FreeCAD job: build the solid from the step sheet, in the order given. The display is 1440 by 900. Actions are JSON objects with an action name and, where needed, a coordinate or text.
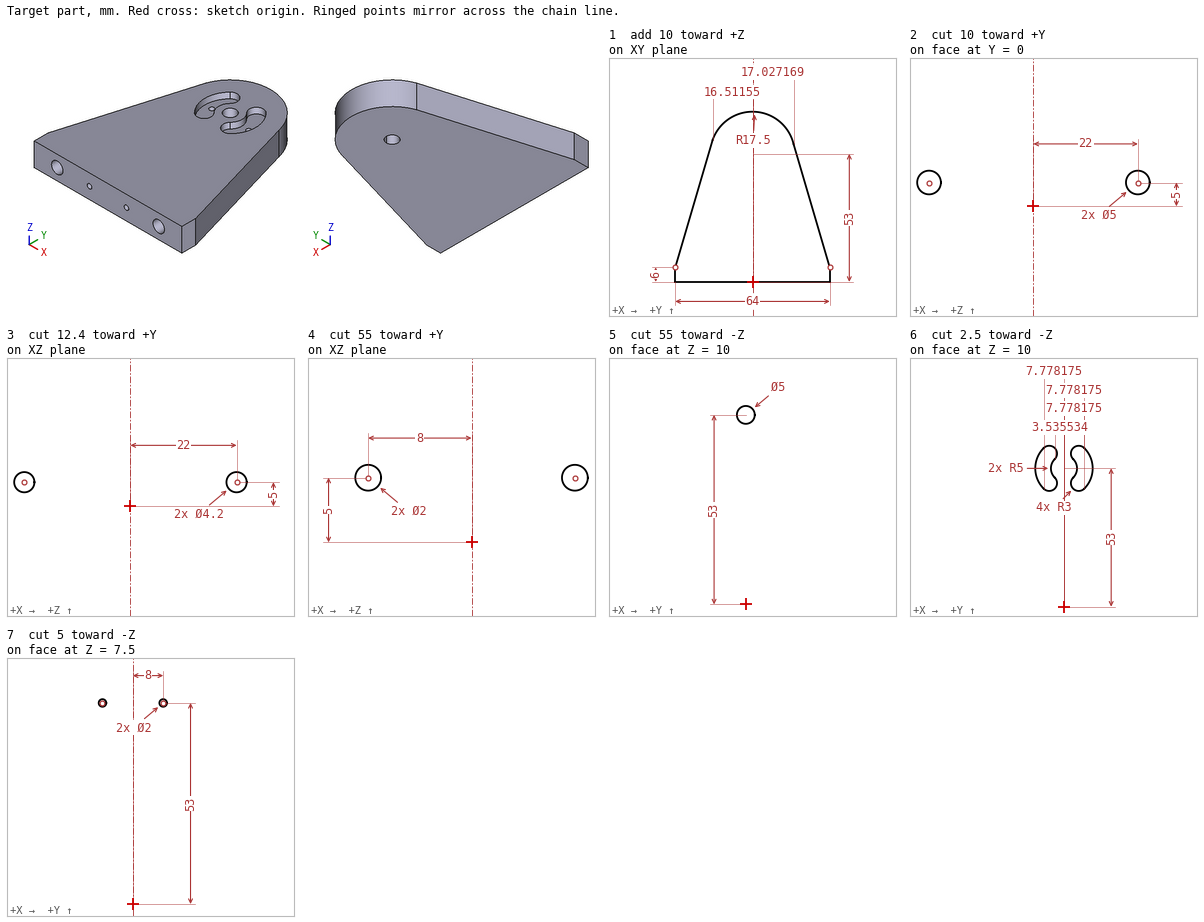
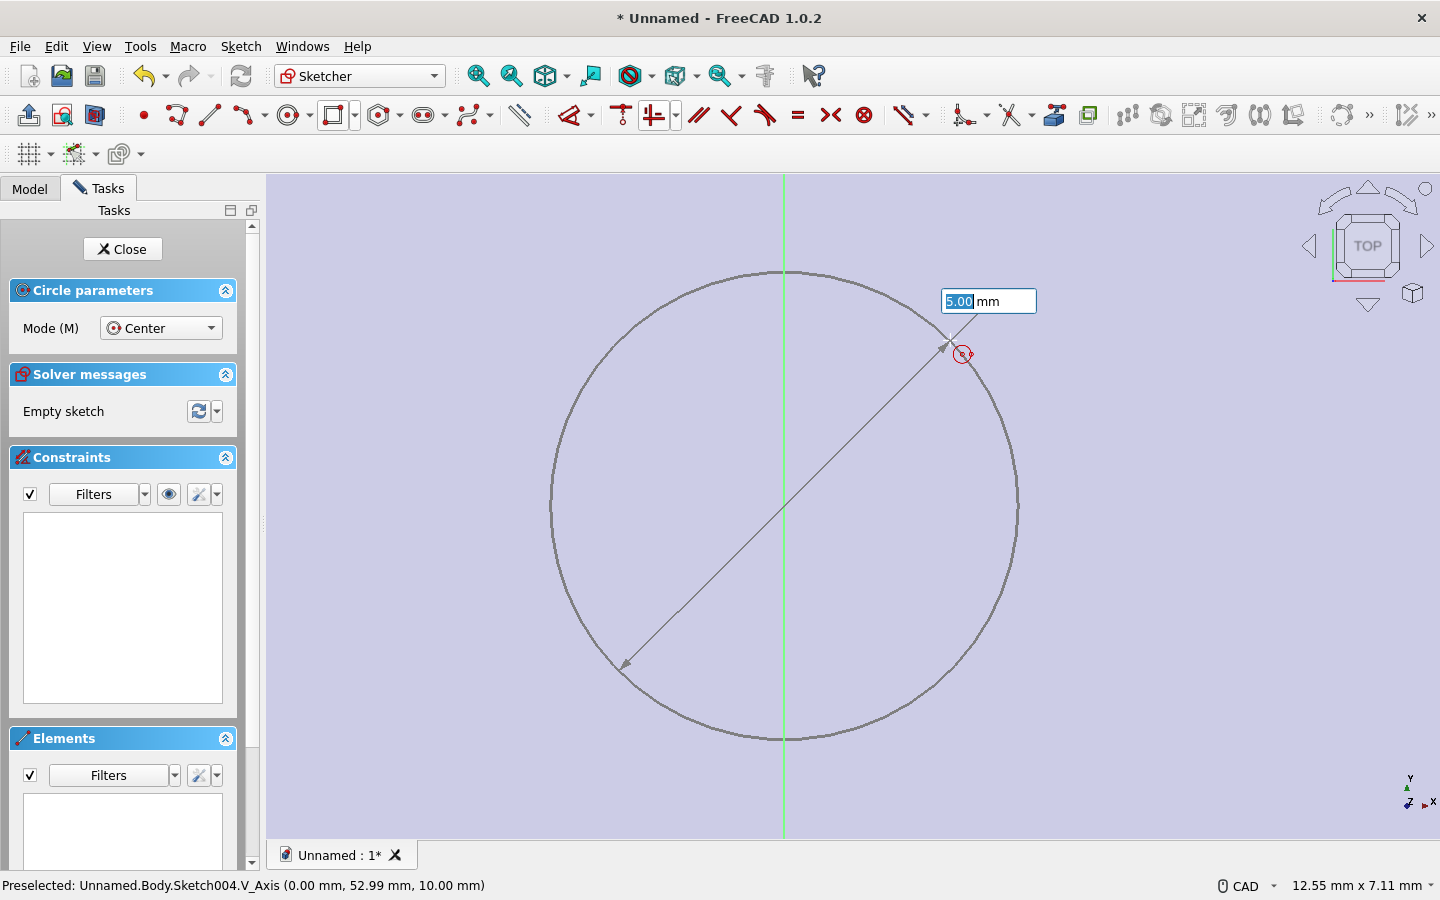
{"action": "type", "text": "5"}
{"action": "key", "text": "Return"}
{"action": "key", "text": "Escape"}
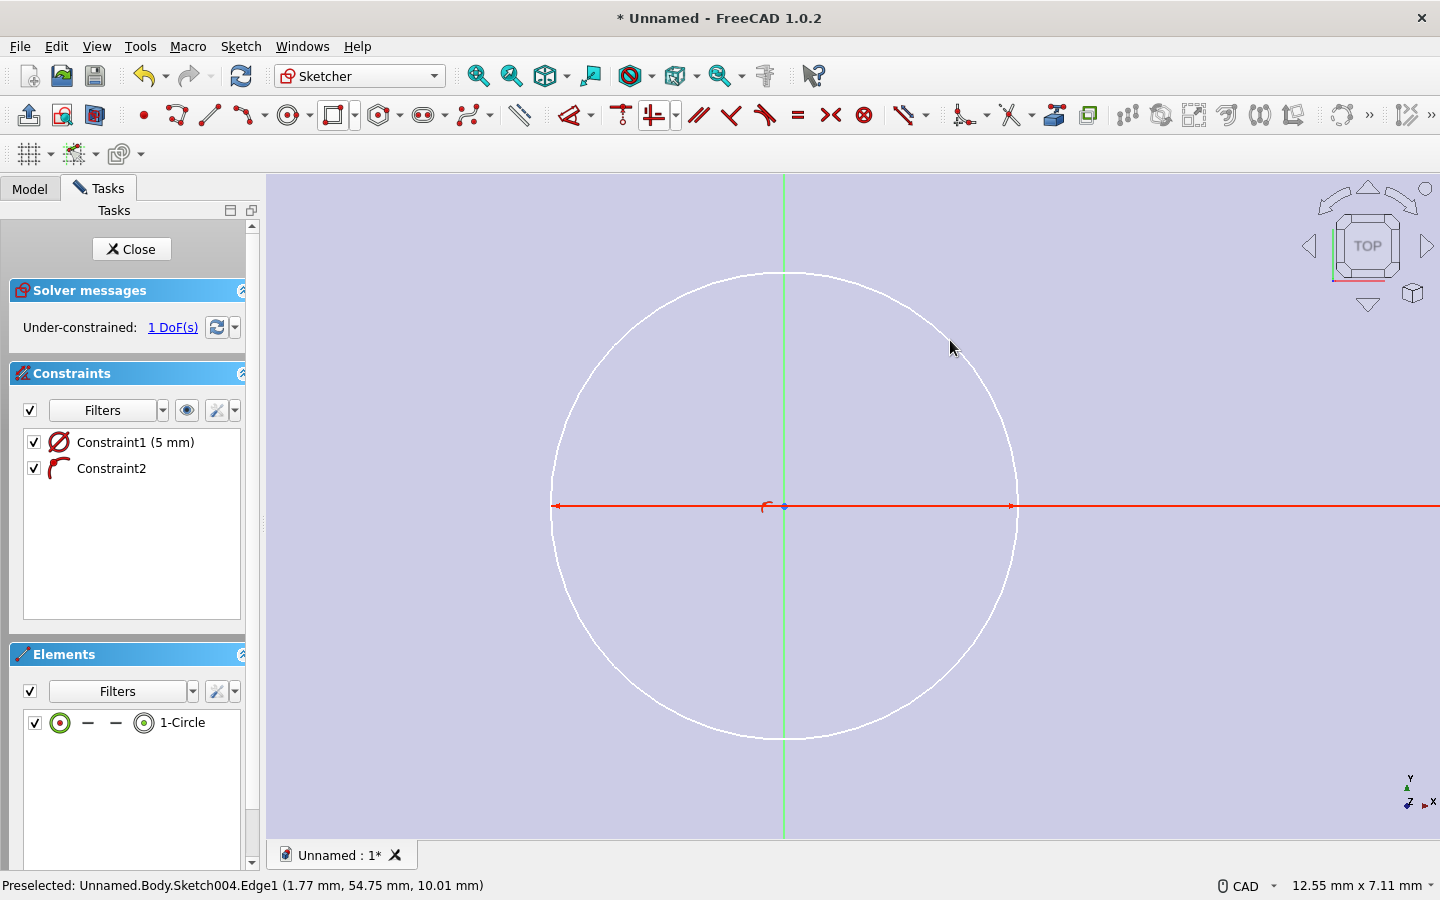
{"action": "left_click", "coordinate": [568, 116]}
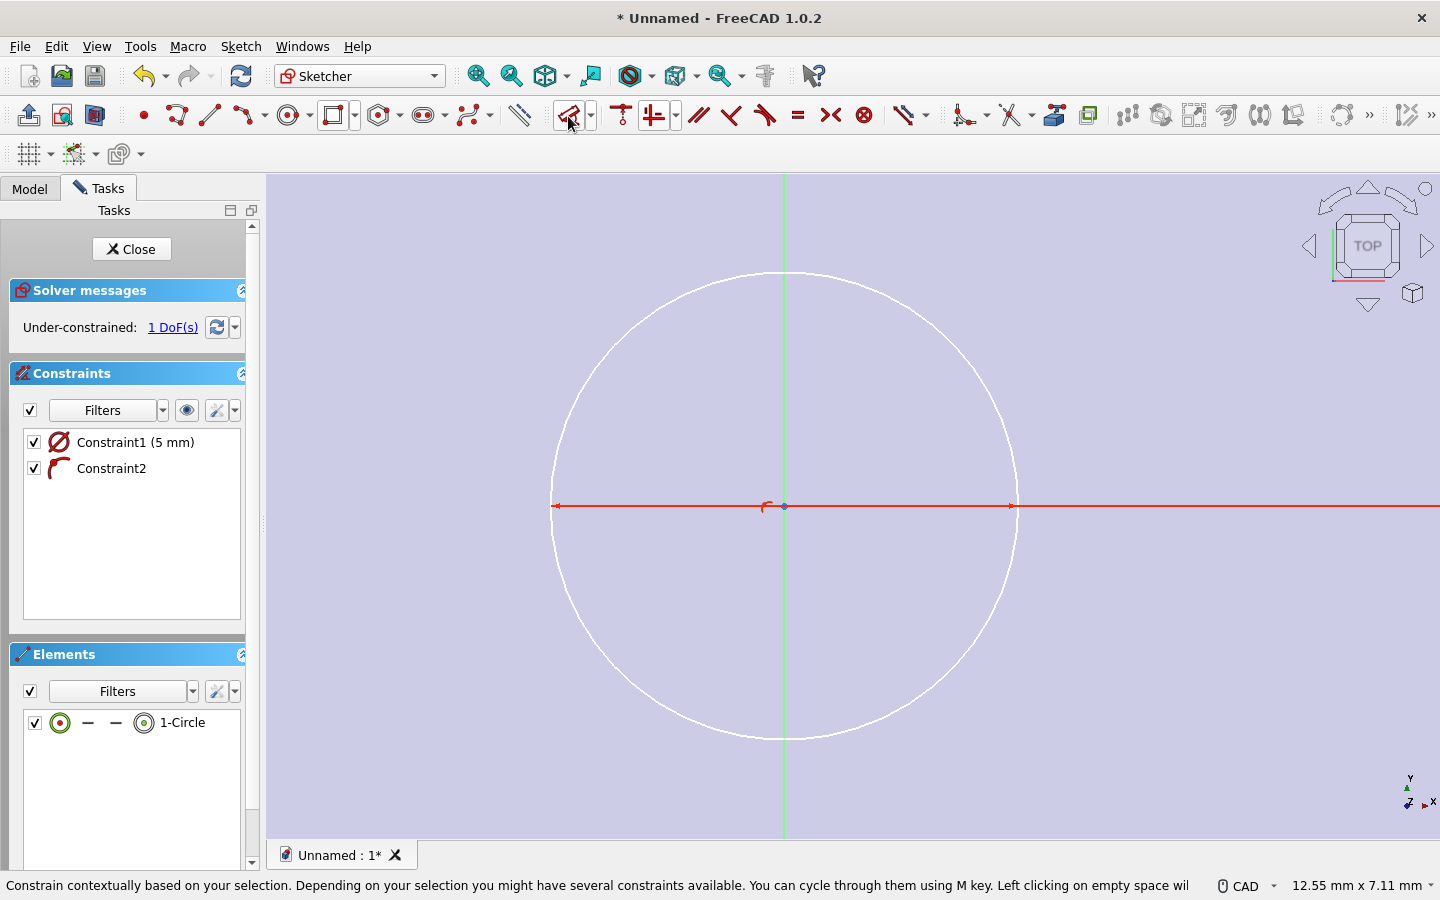
{"action": "left_click", "coordinate": [784, 506]}
{"action": "left_click", "coordinate": [818, 659]}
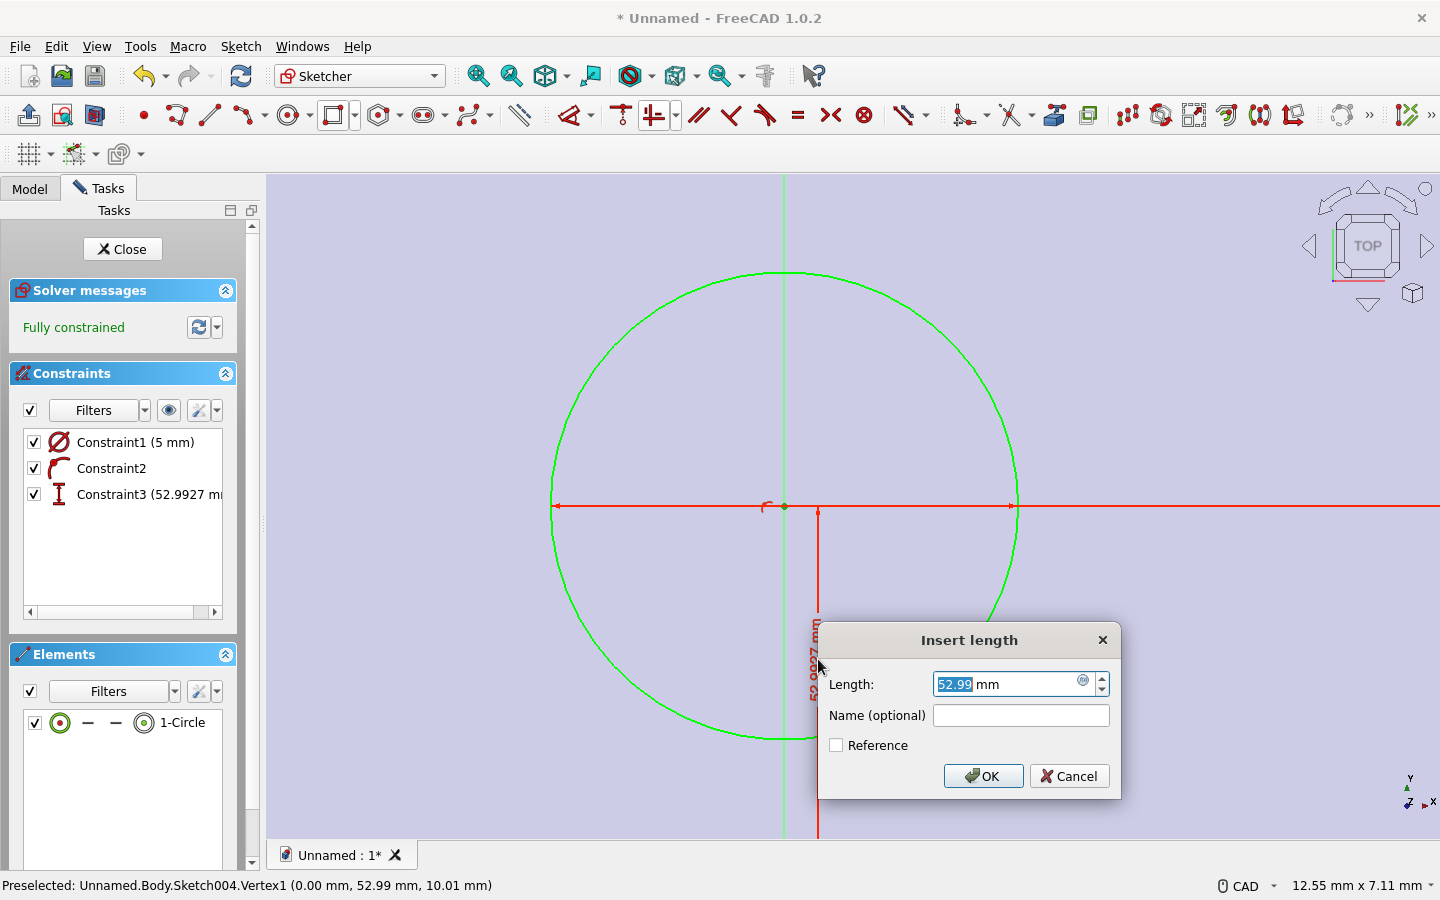
{"action": "type", "text": "53"}
{"action": "key", "text": "Return"}
{"action": "key", "text": "Escape"}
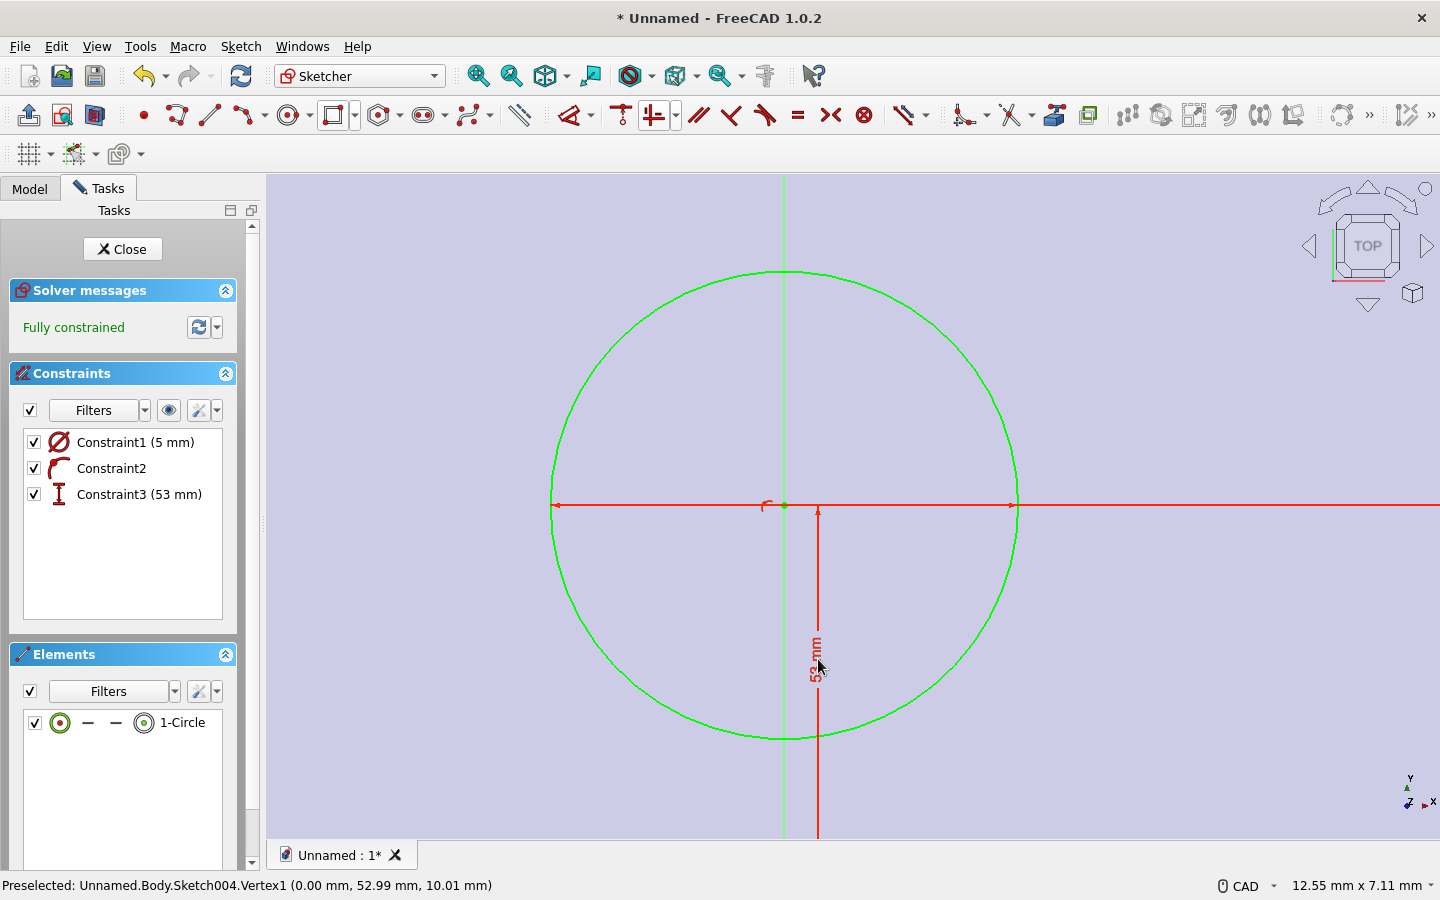
{"action": "left_click", "coordinate": [123, 249]}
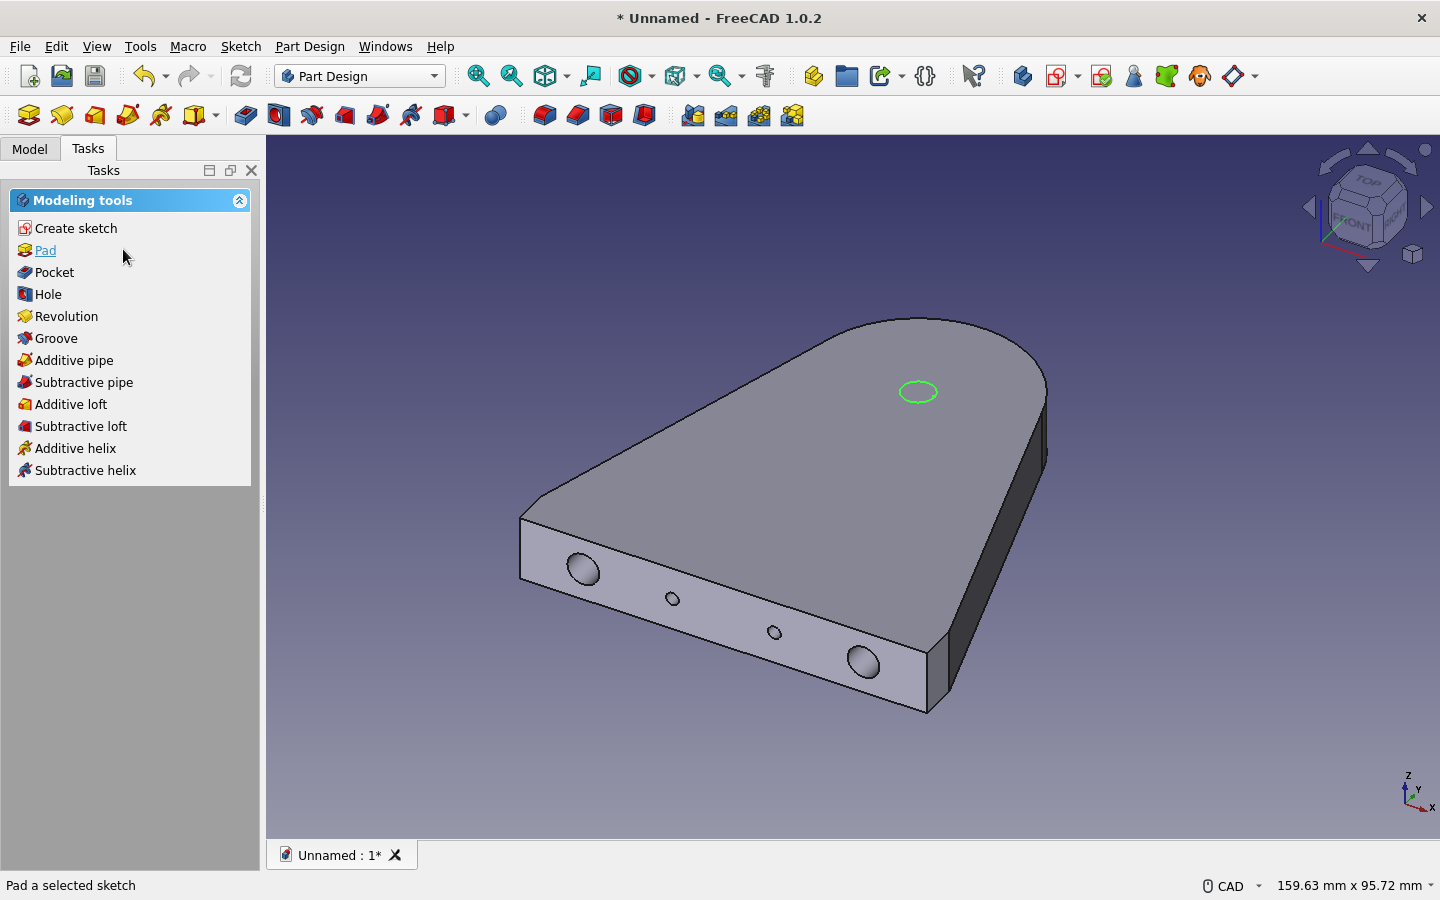
{"action": "left_click", "coordinate": [246, 116]}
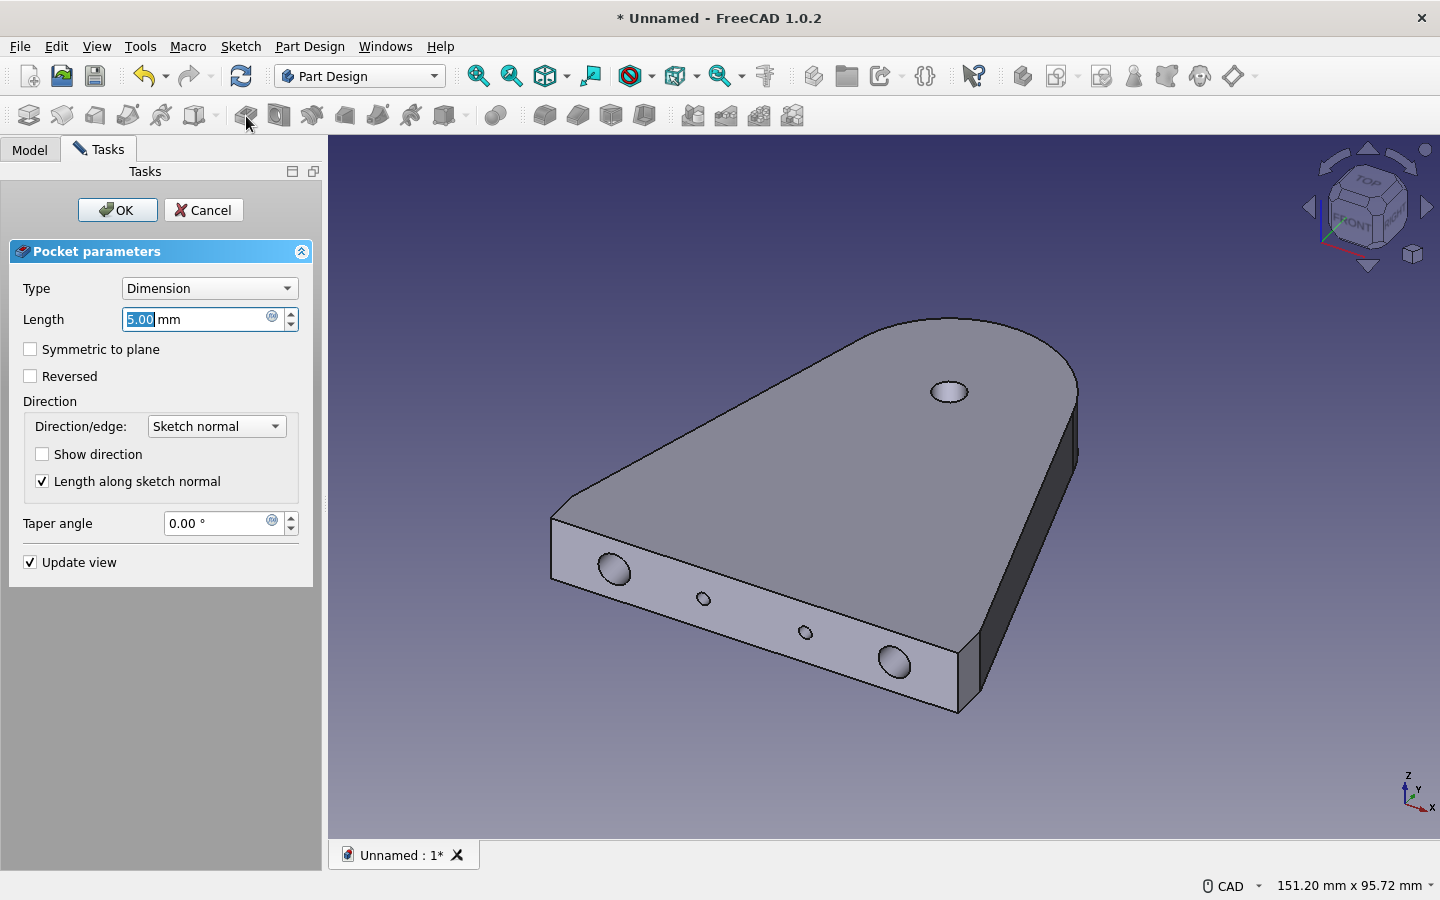
{"action": "type", "text": "55"}
{"action": "key", "text": "Tab"}